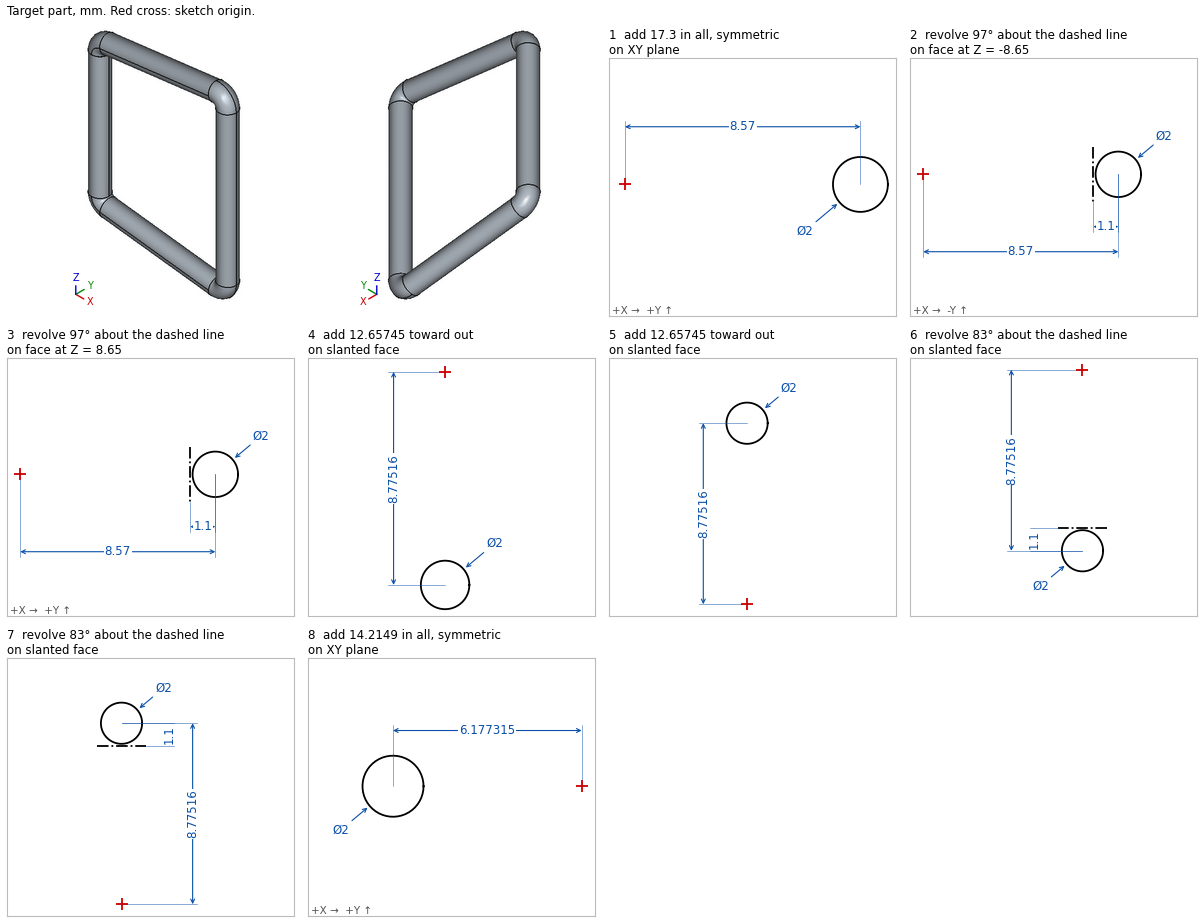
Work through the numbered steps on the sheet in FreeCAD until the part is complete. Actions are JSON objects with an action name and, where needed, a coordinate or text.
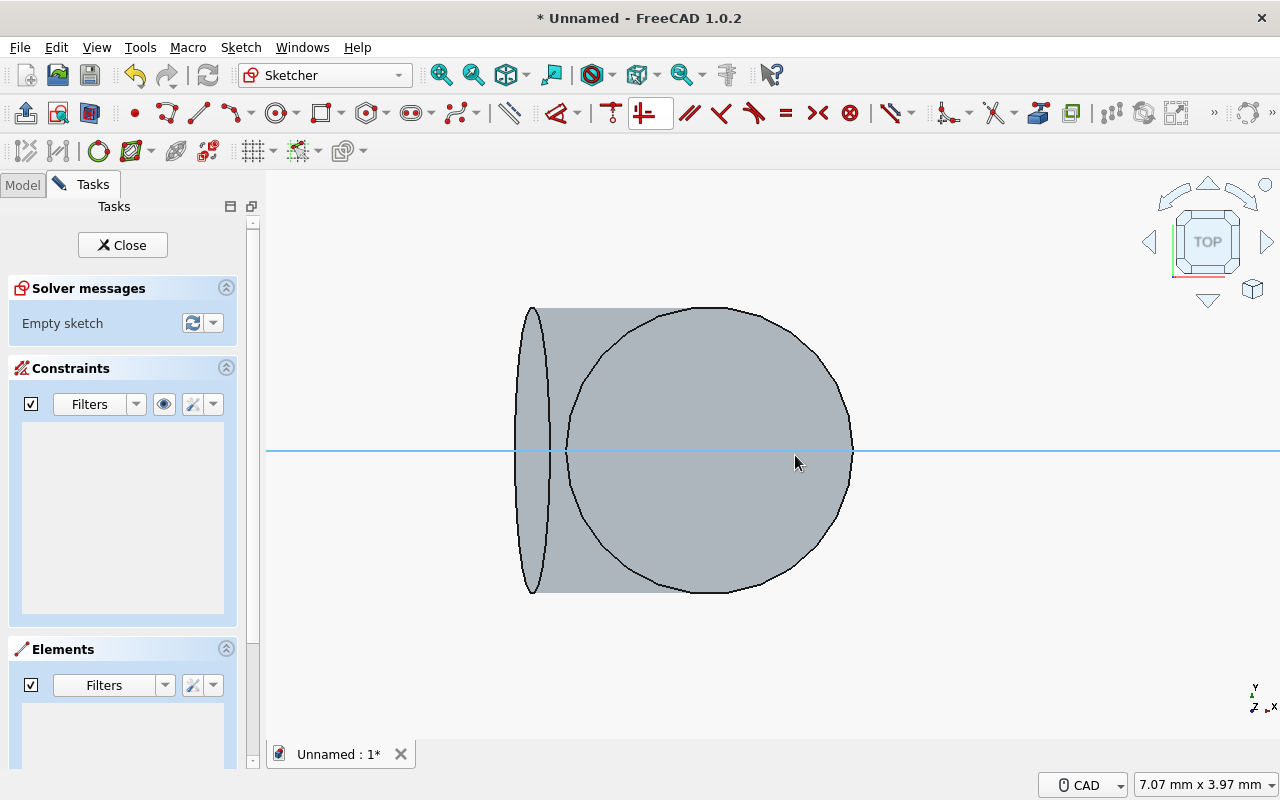
{"action": "key", "text": "g c"}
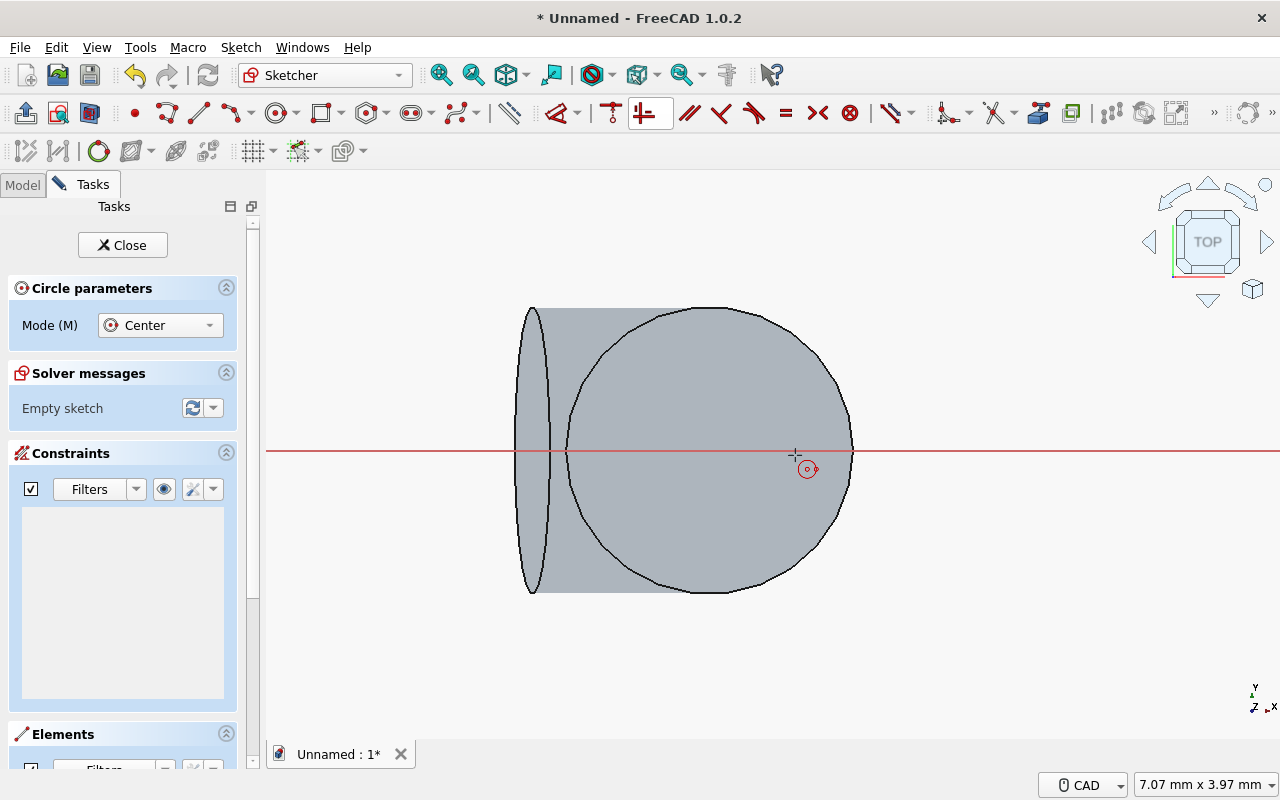
{"action": "left_click", "coordinate": [710, 451]}
{"action": "mouse_move", "coordinate": [811, 349]}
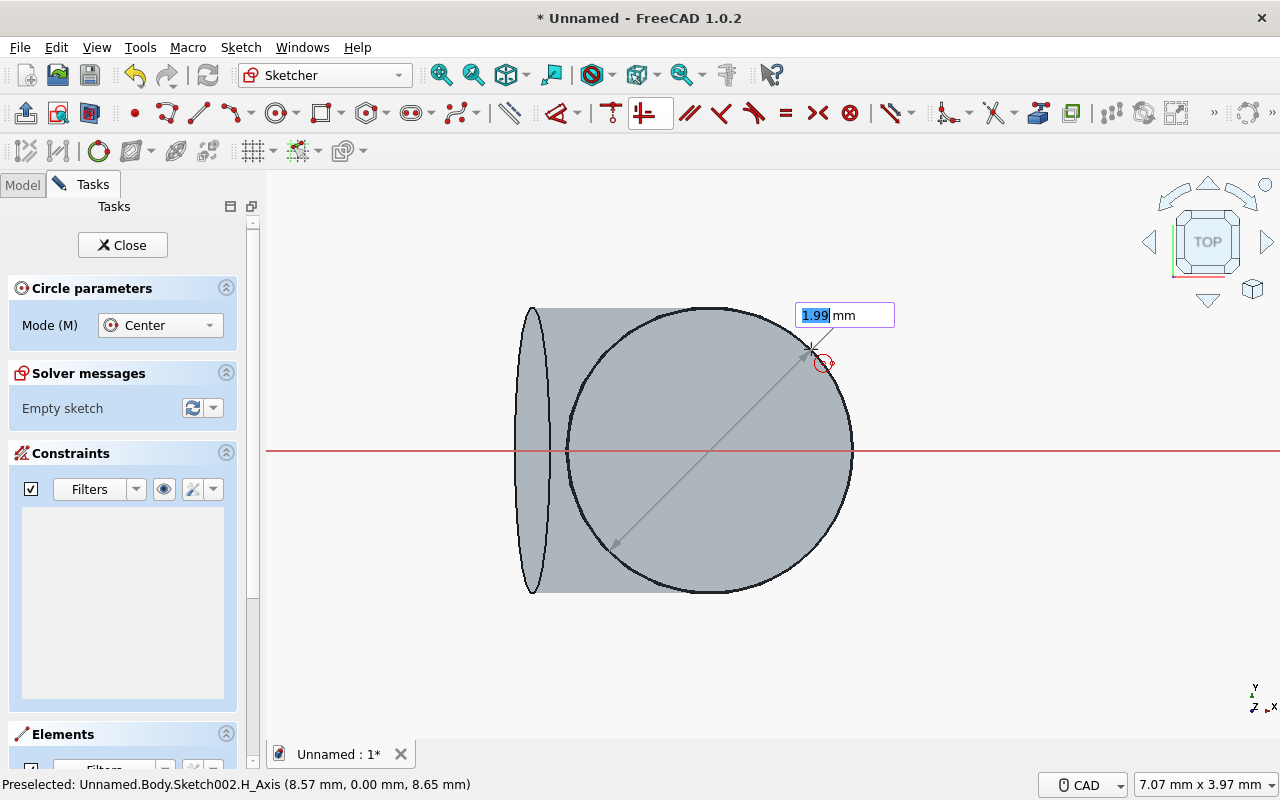
{"action": "type", "text": "2"}
{"action": "key", "text": "Return"}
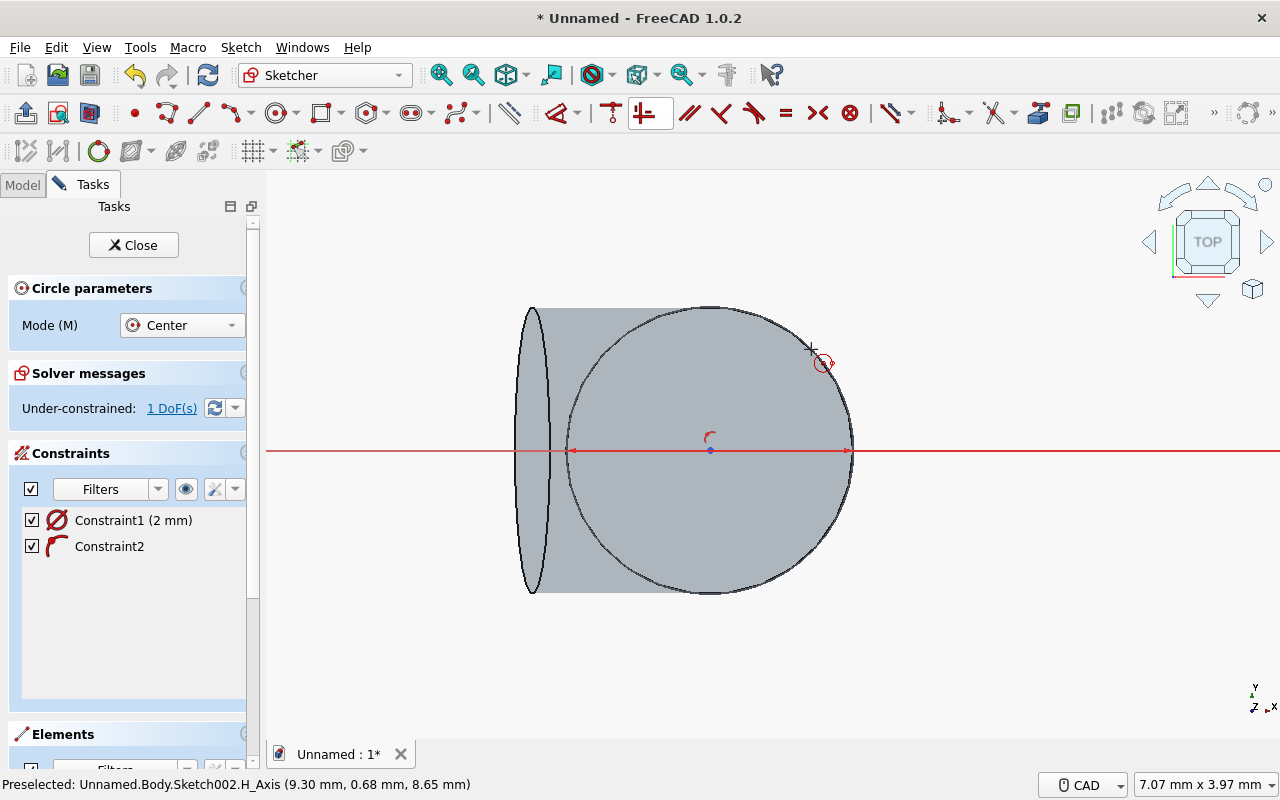
{"action": "key", "text": "g l"}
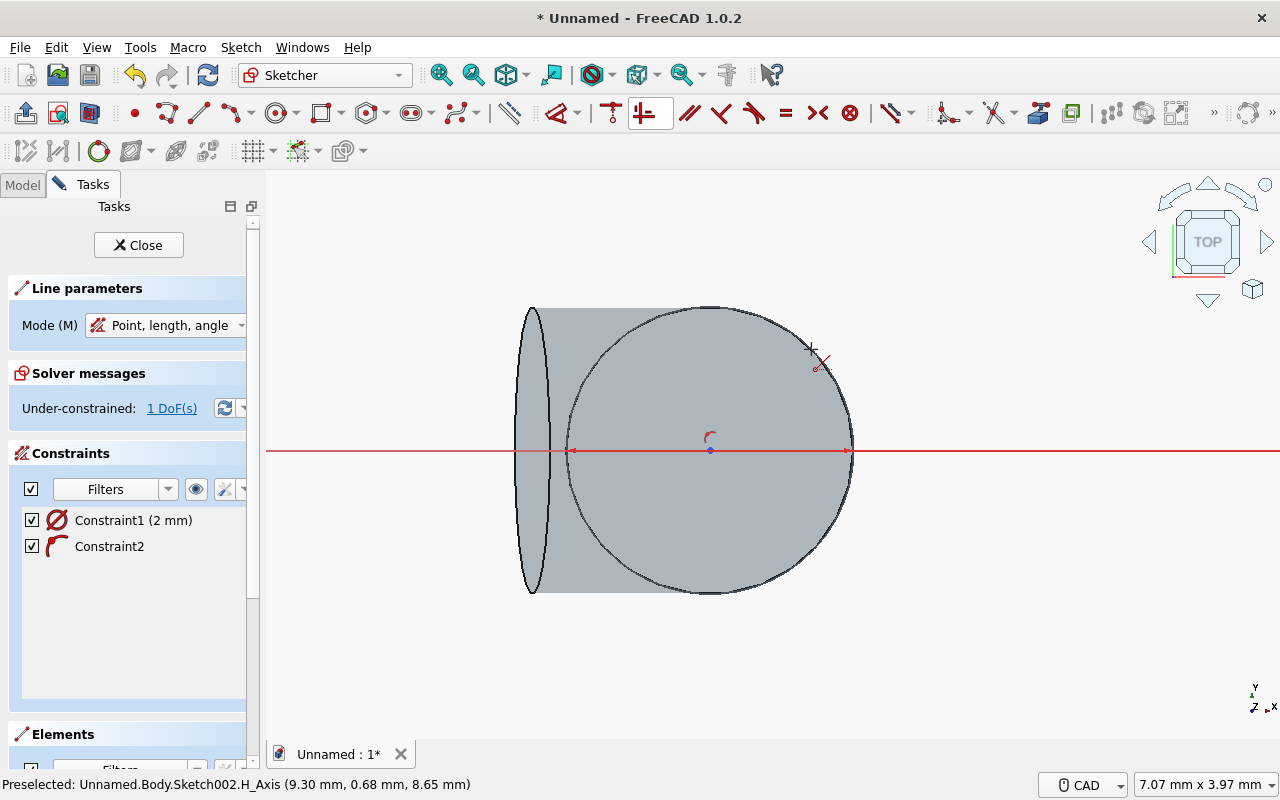
{"action": "left_click", "coordinate": [552, 278]}
{"action": "left_click", "coordinate": [552, 623]}
{"action": "key", "text": "Escape"}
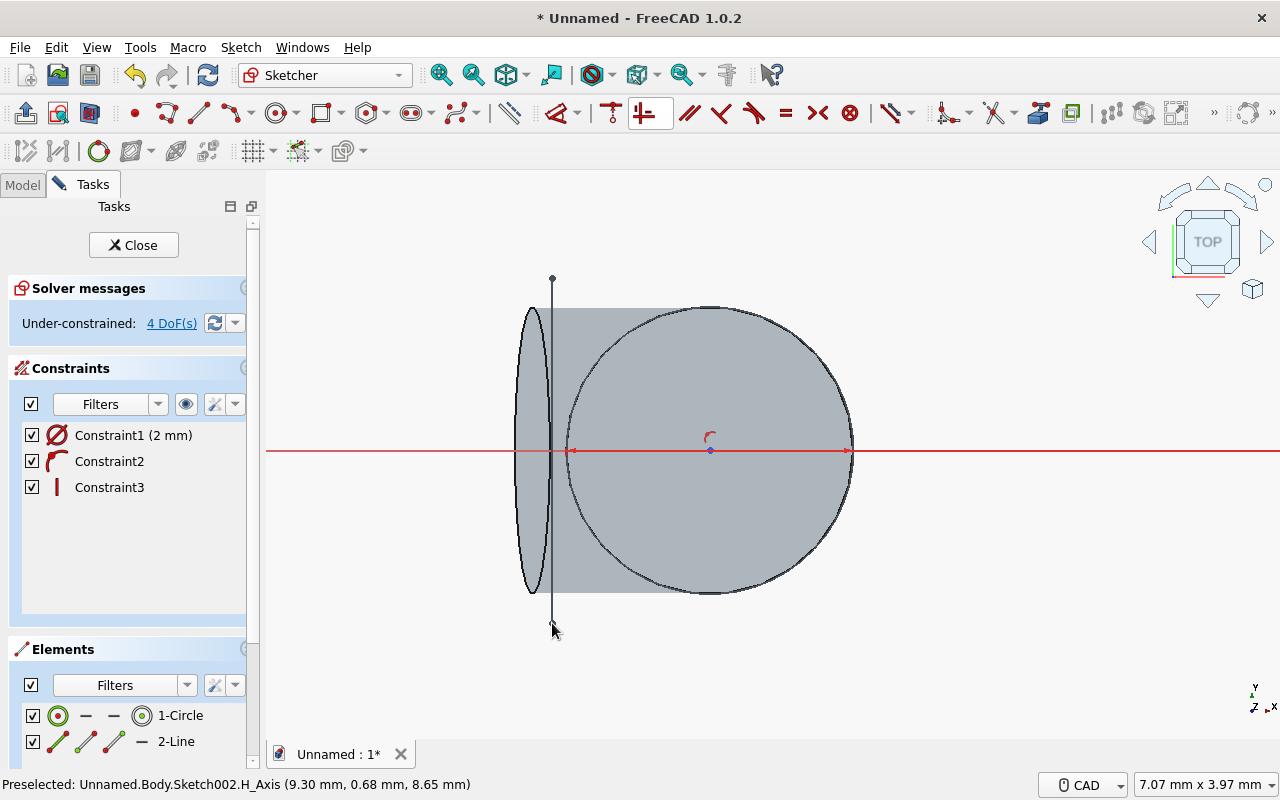
{"action": "left_click", "coordinate": [552, 383]}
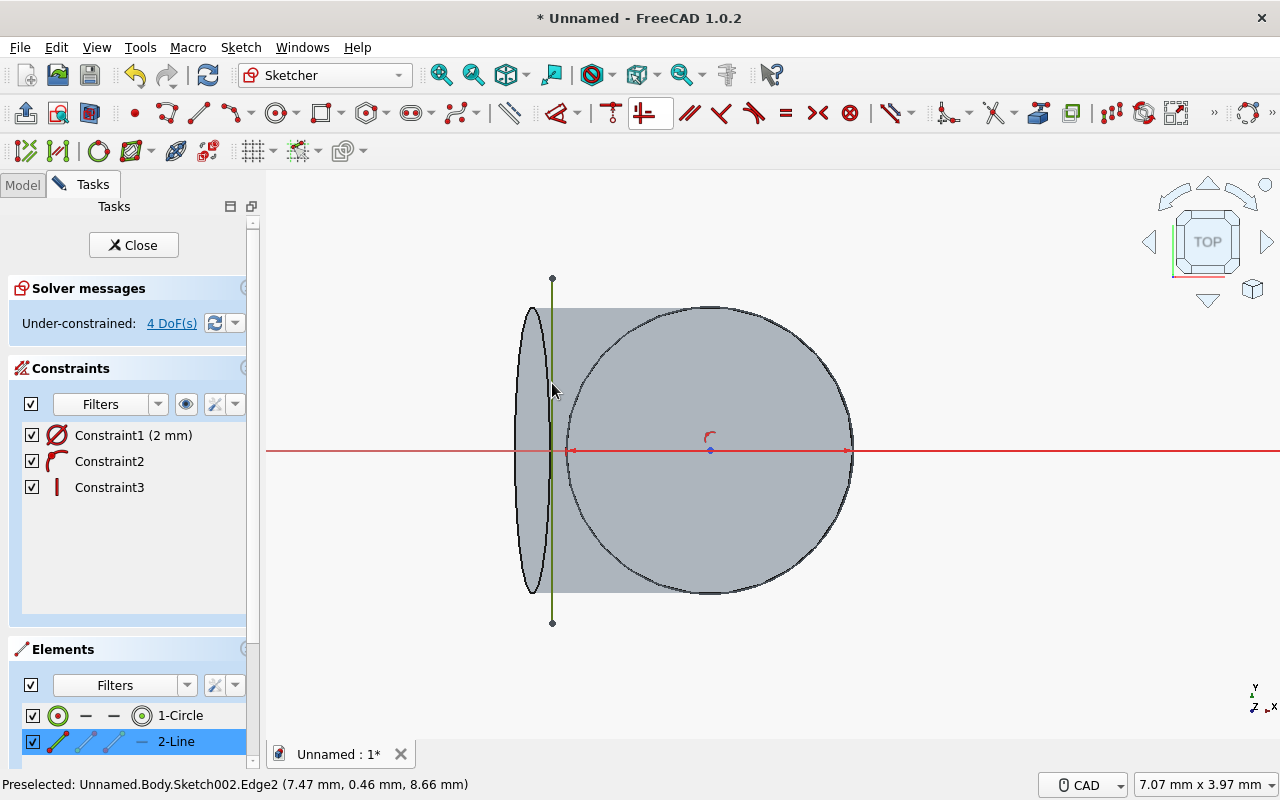
{"action": "left_click", "coordinate": [510, 114]}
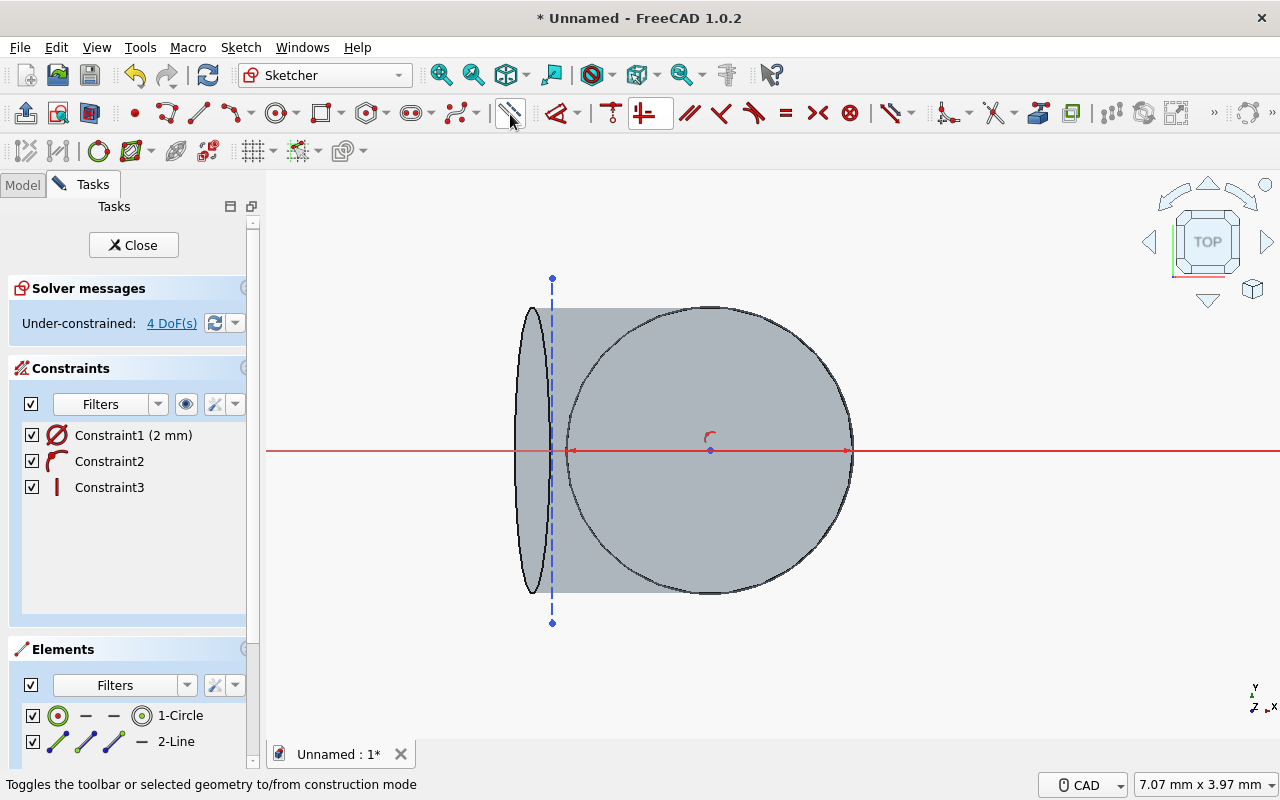
{"action": "left_click", "coordinate": [556, 114]}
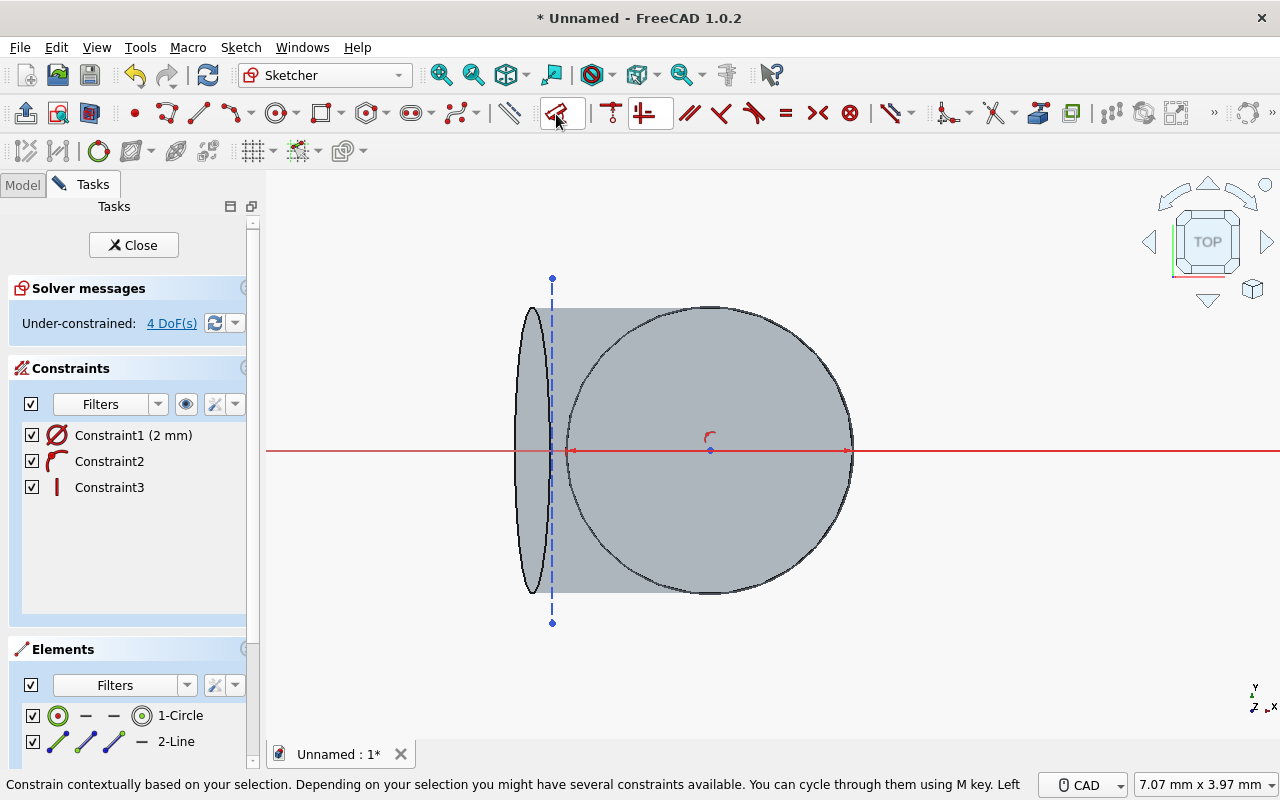
{"action": "left_click", "coordinate": [712, 453]}
{"action": "left_click", "coordinate": [502, 485]}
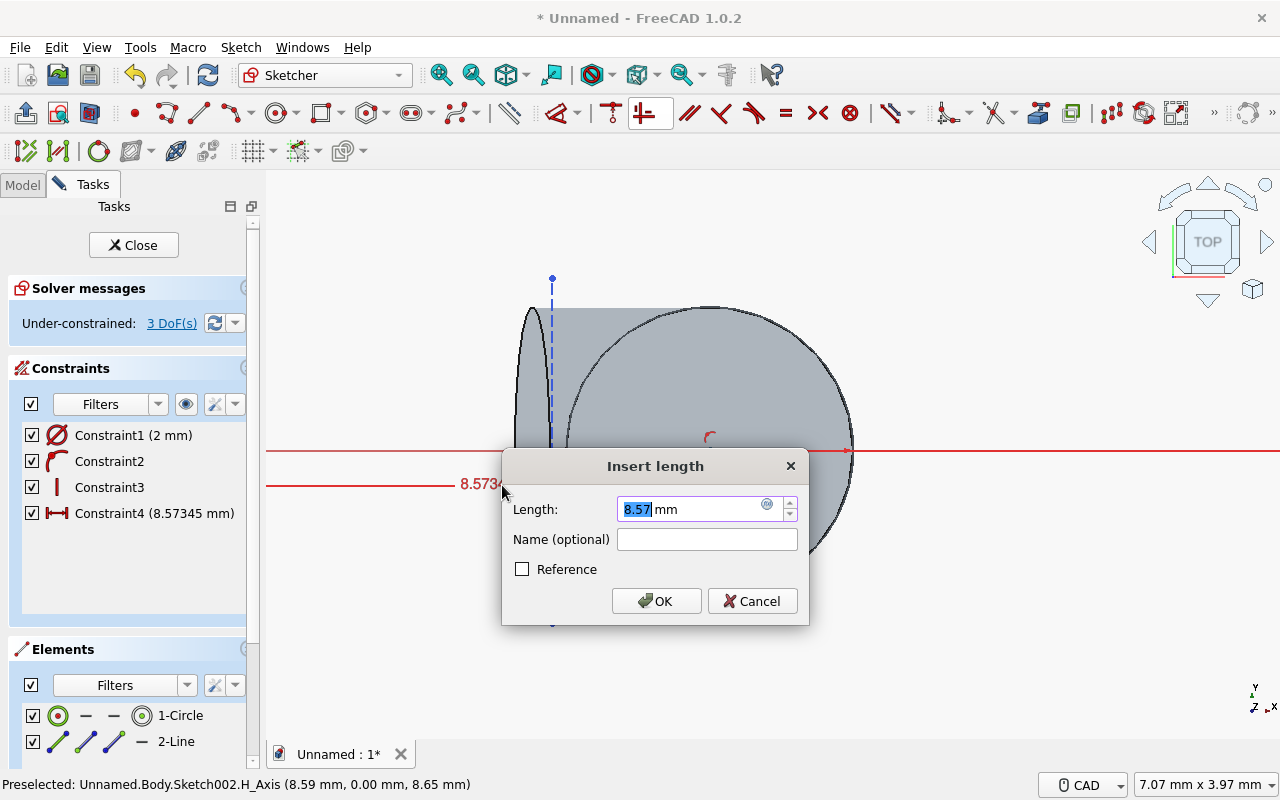
{"action": "type", "text": "8.57"}
{"action": "key", "text": "Return"}